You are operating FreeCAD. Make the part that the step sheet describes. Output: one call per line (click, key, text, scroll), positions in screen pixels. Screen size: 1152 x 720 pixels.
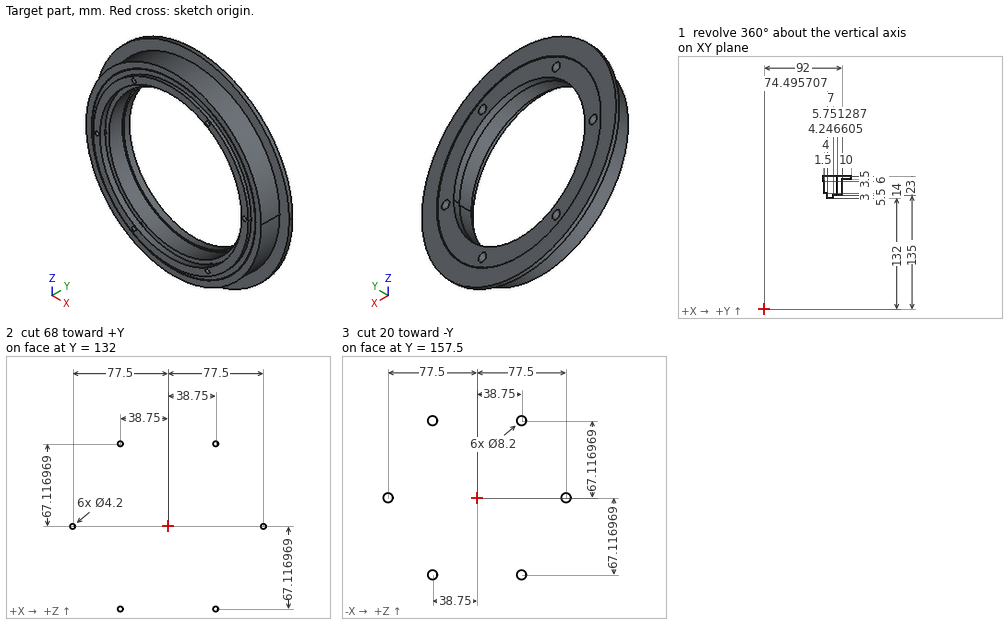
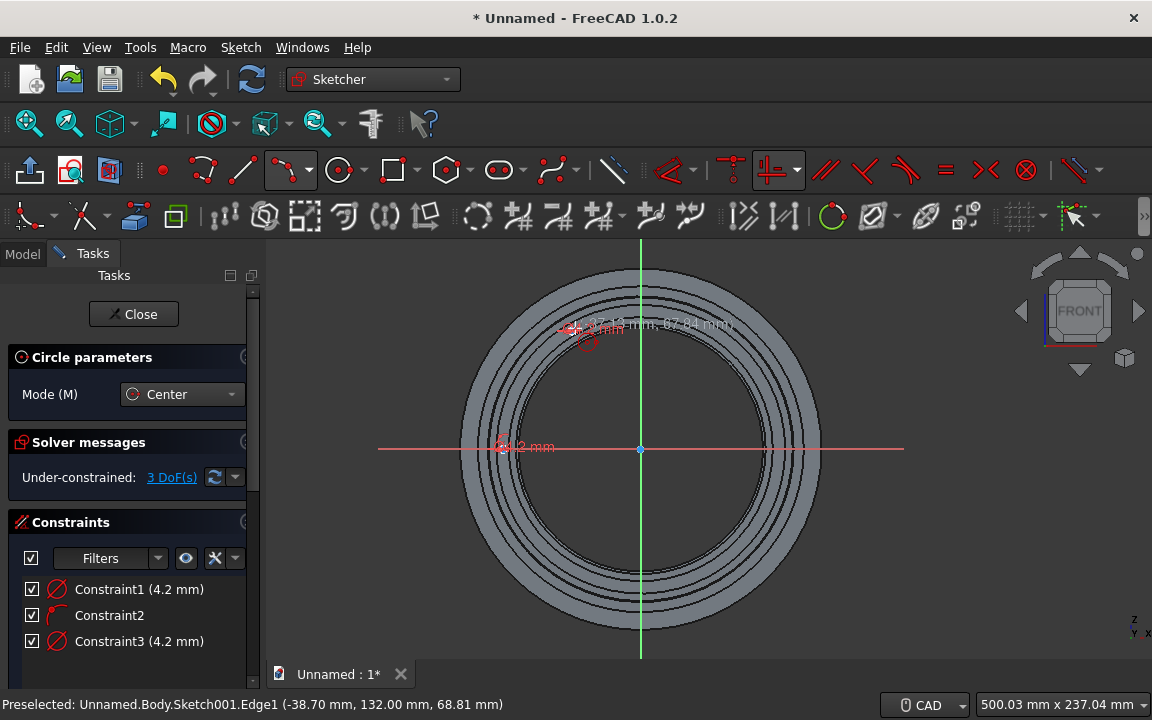
scroll(709, 330, up, 10)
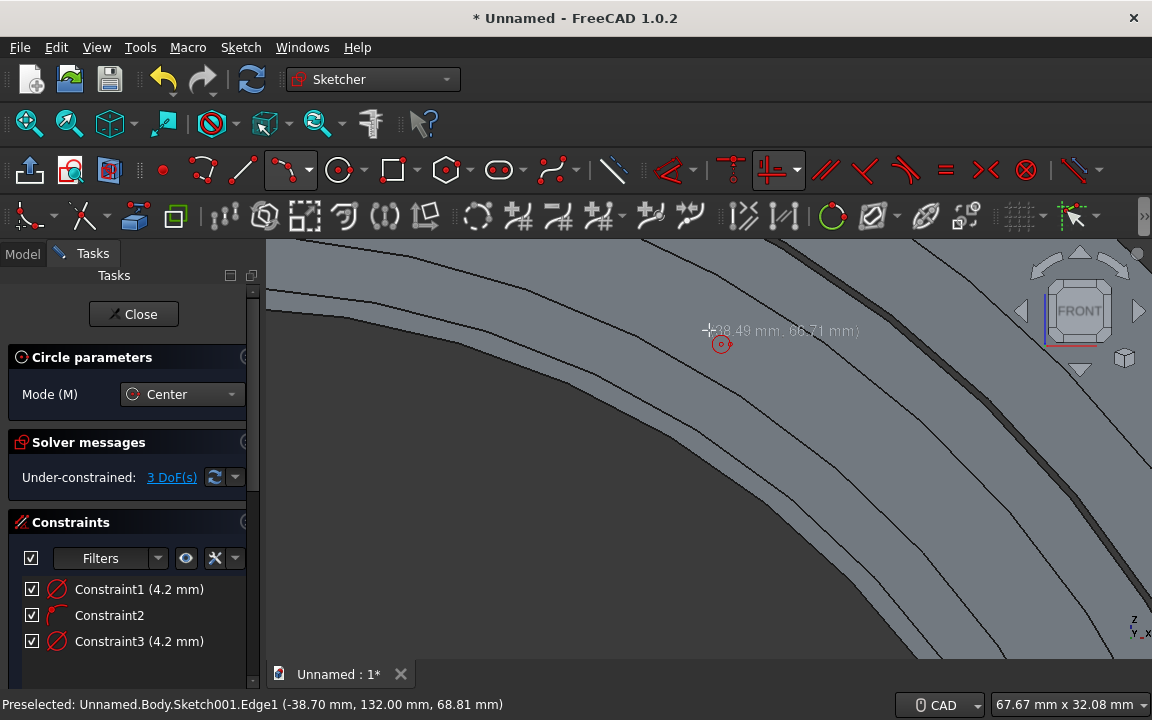
scroll(709, 330, down, 10)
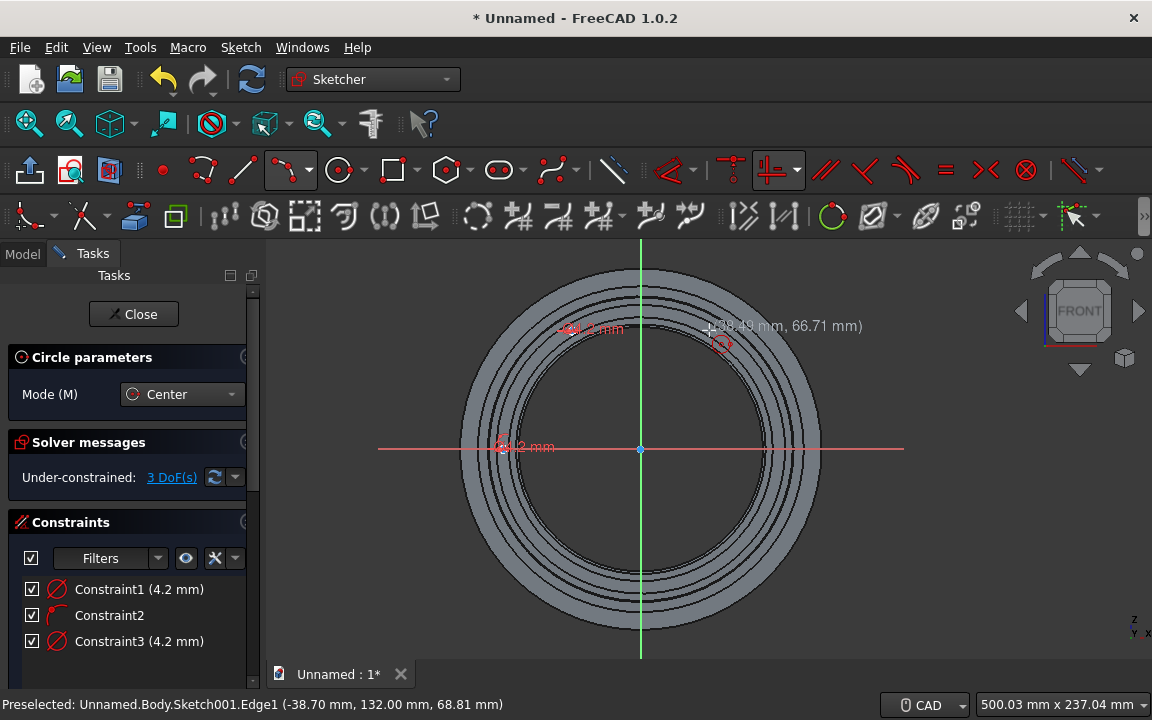
click(709, 330)
move(712, 328)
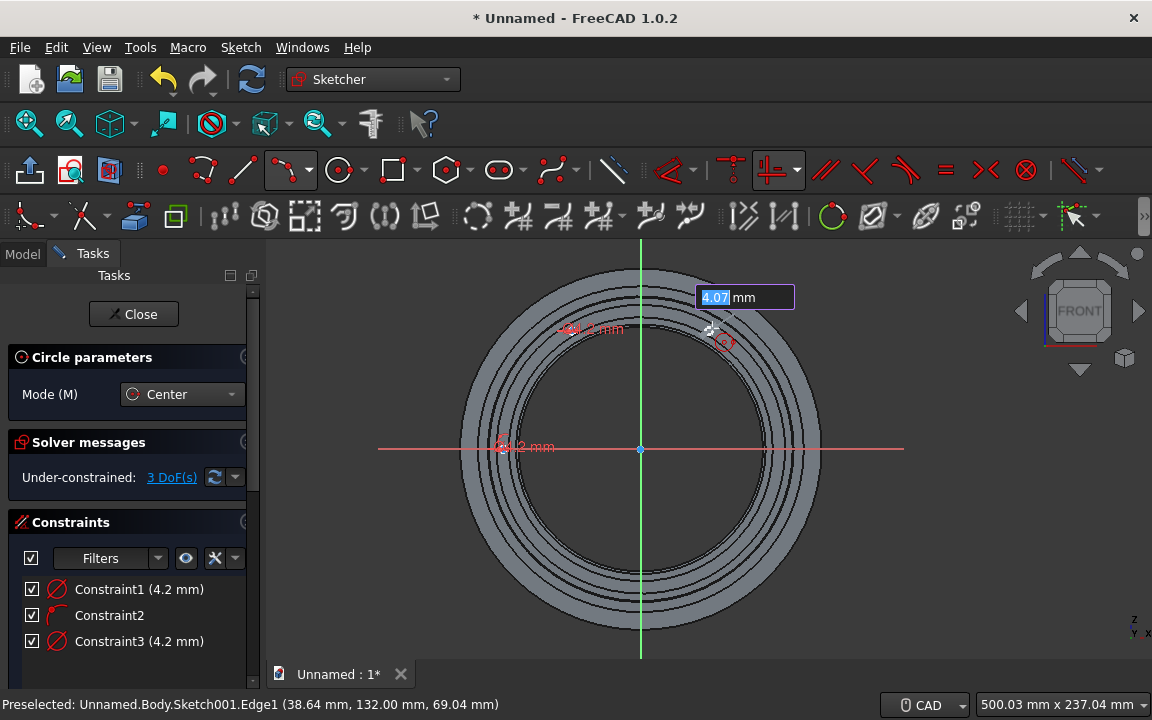
text(4.2)
key(Return)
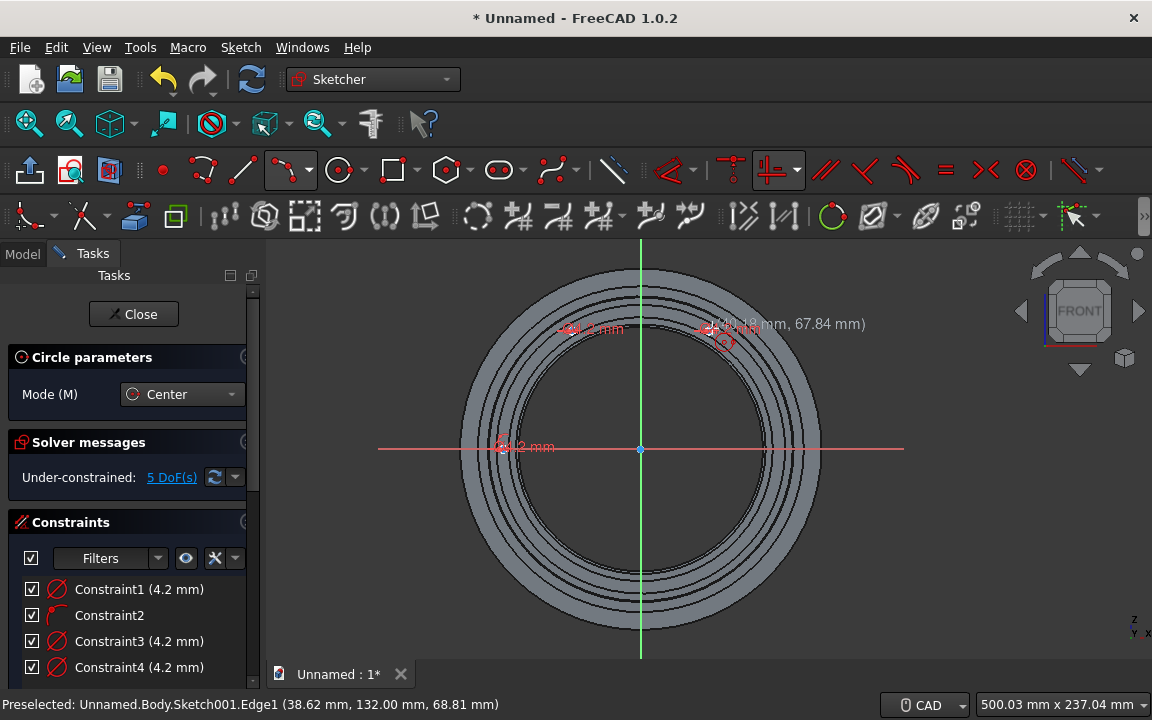
scroll(778, 449, up, 10)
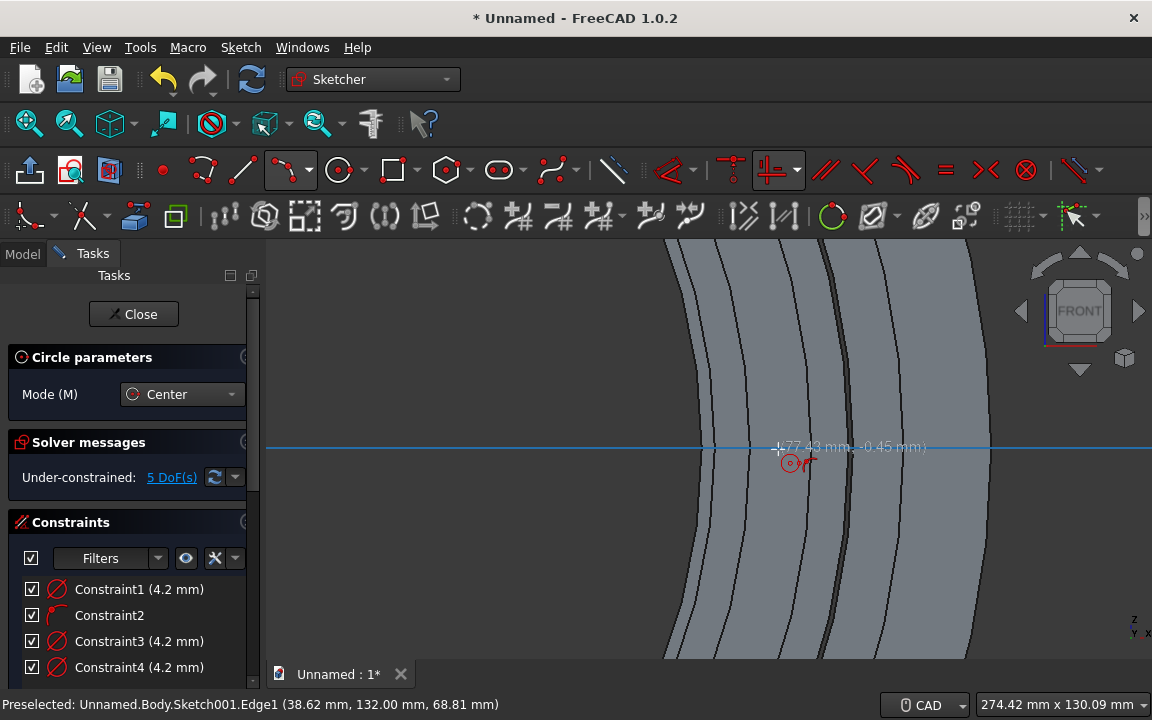
scroll(778, 449, down, 10)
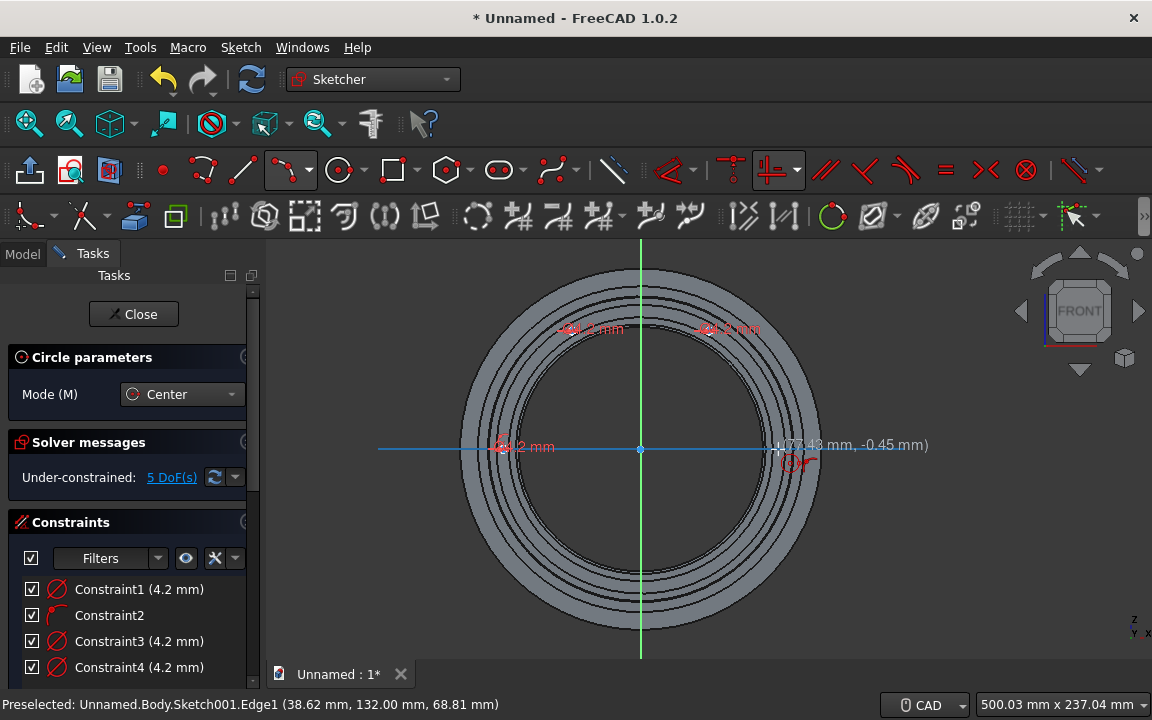
click(778, 449)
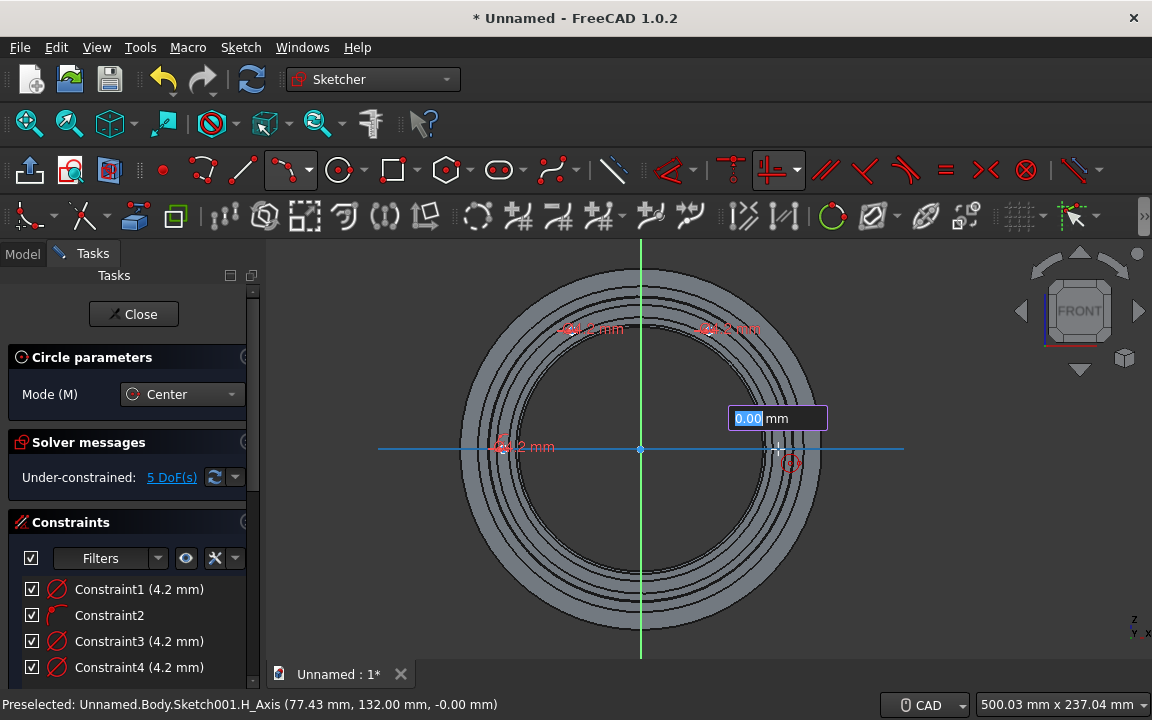
scroll(777, 453, up, 8)
move(774, 450)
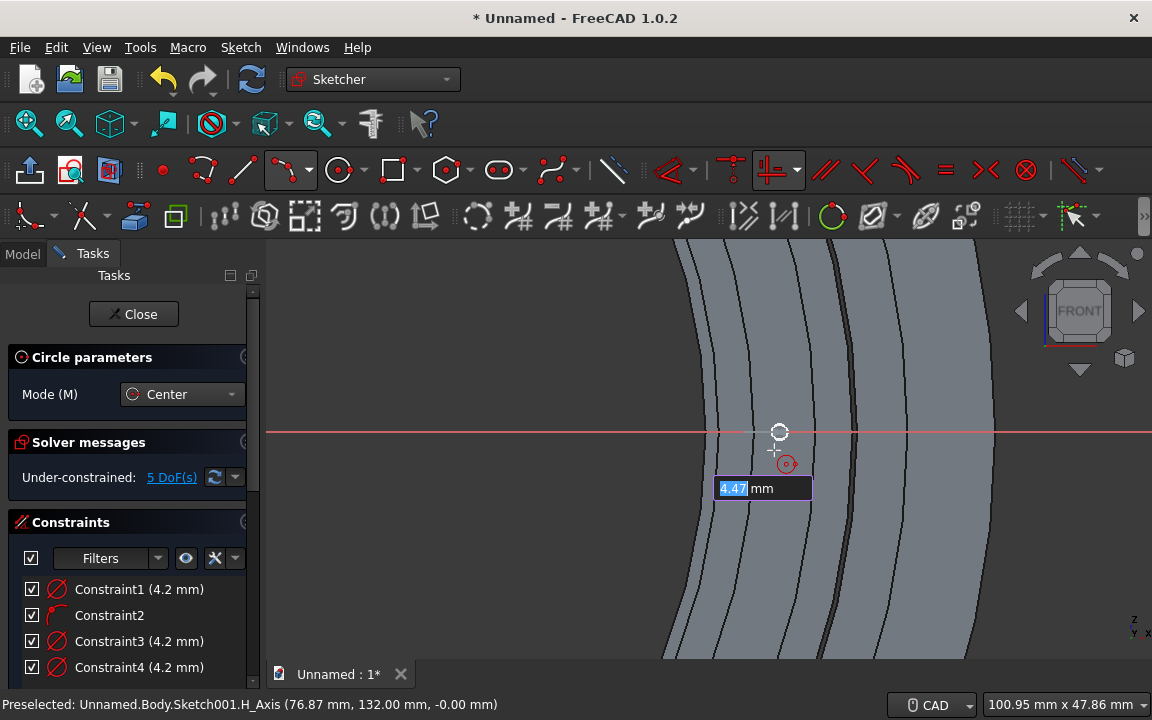
text(4.2)
key(Return)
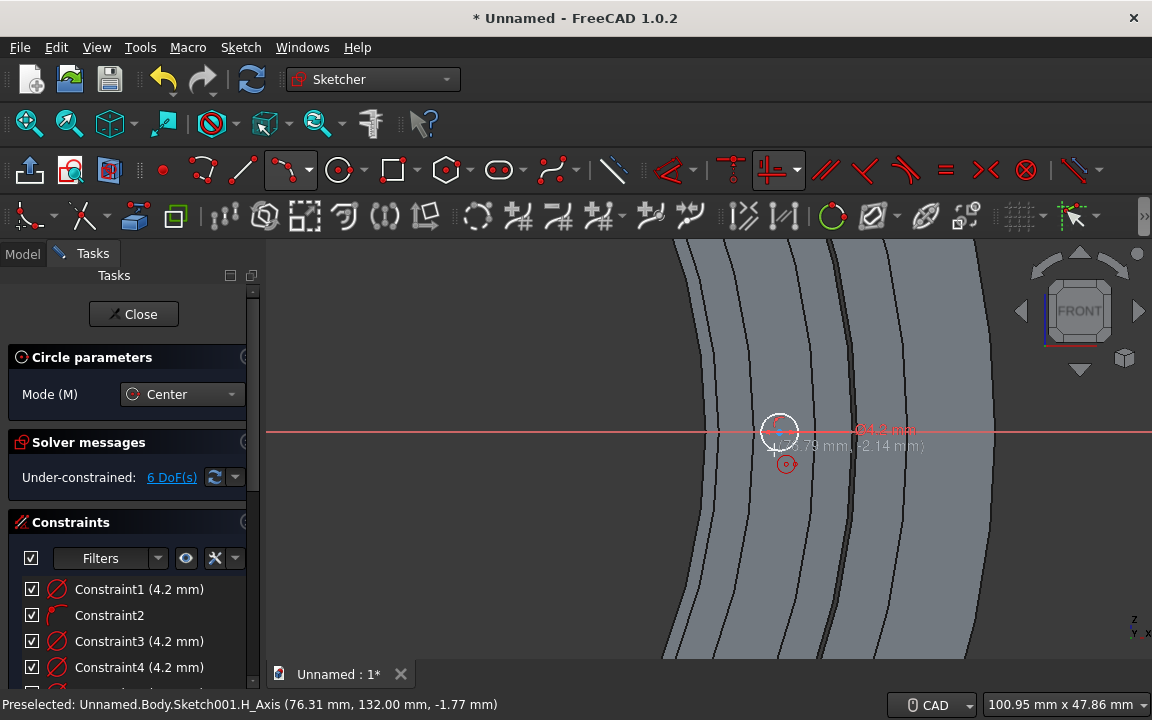
scroll(777, 453, down, 8)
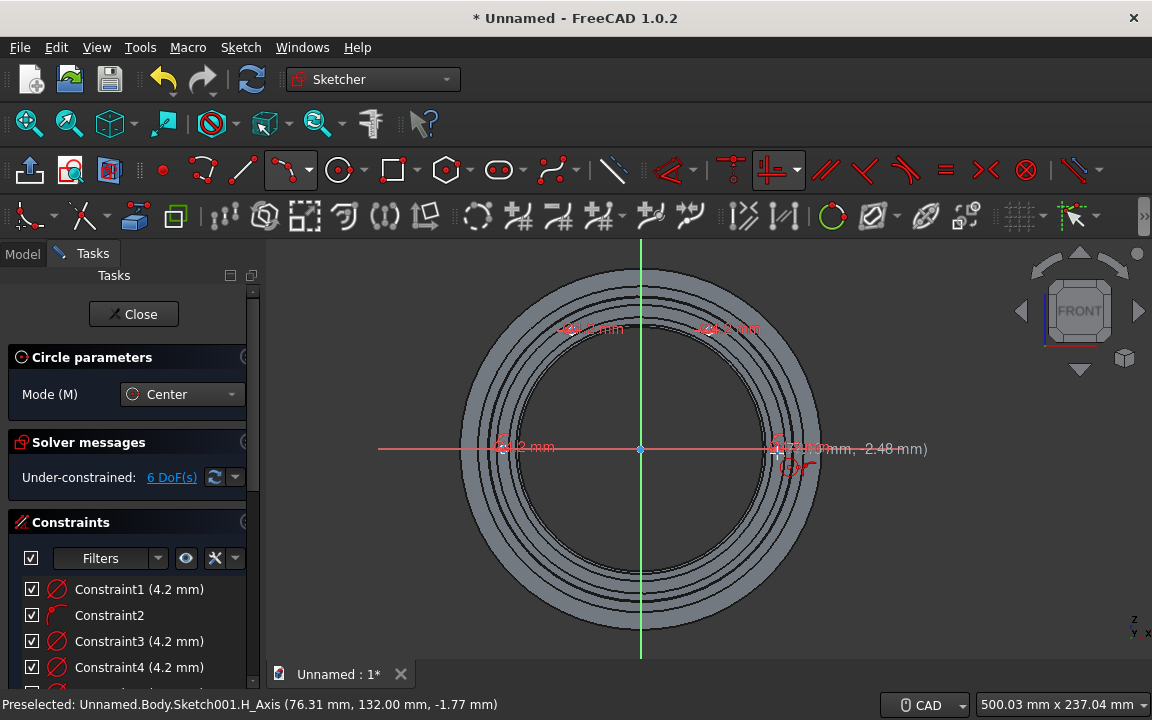
scroll(709, 568, up, 10)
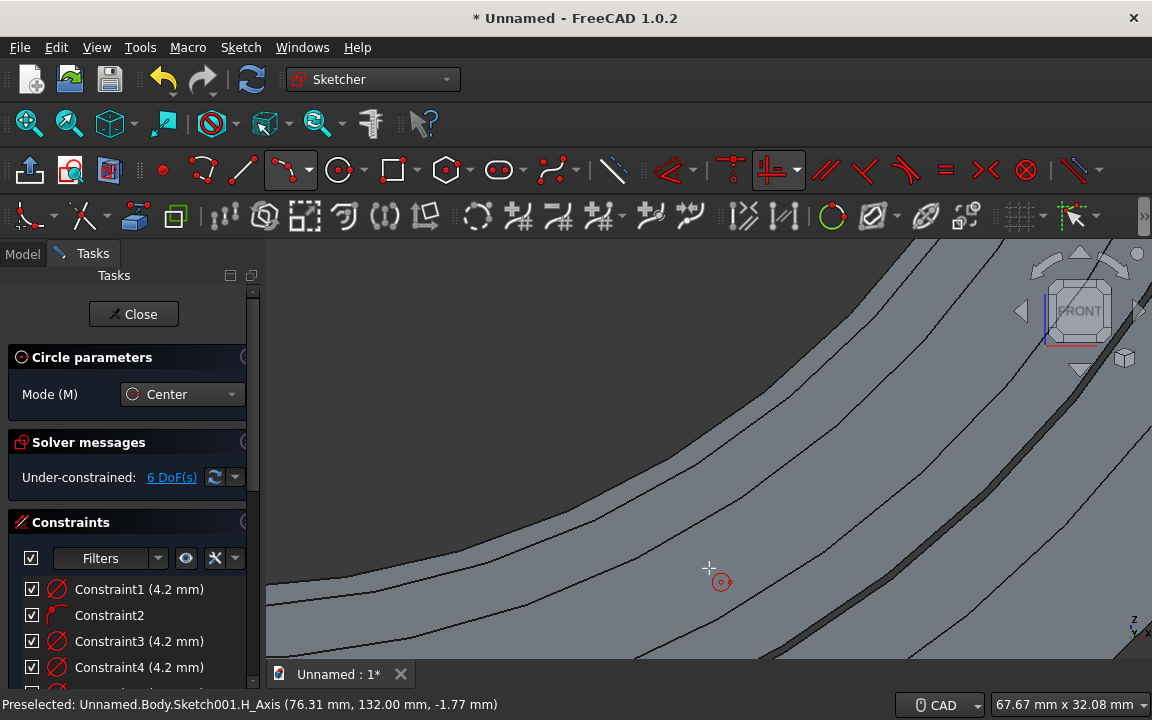
scroll(709, 569, down, 10)